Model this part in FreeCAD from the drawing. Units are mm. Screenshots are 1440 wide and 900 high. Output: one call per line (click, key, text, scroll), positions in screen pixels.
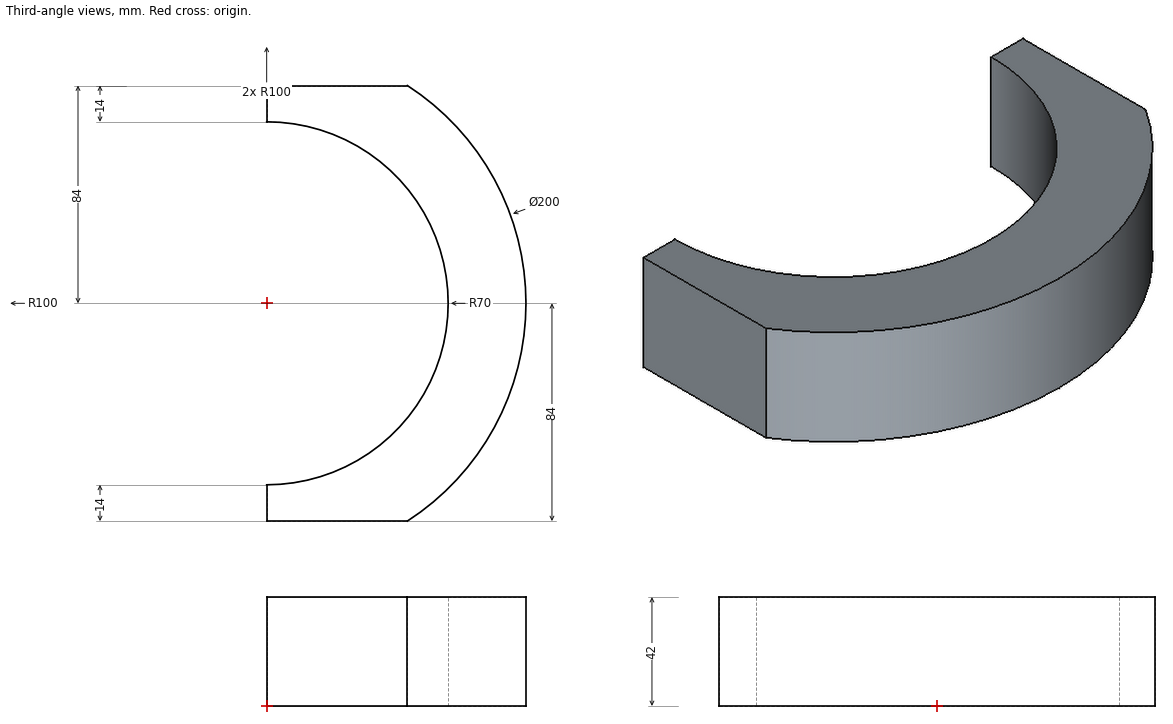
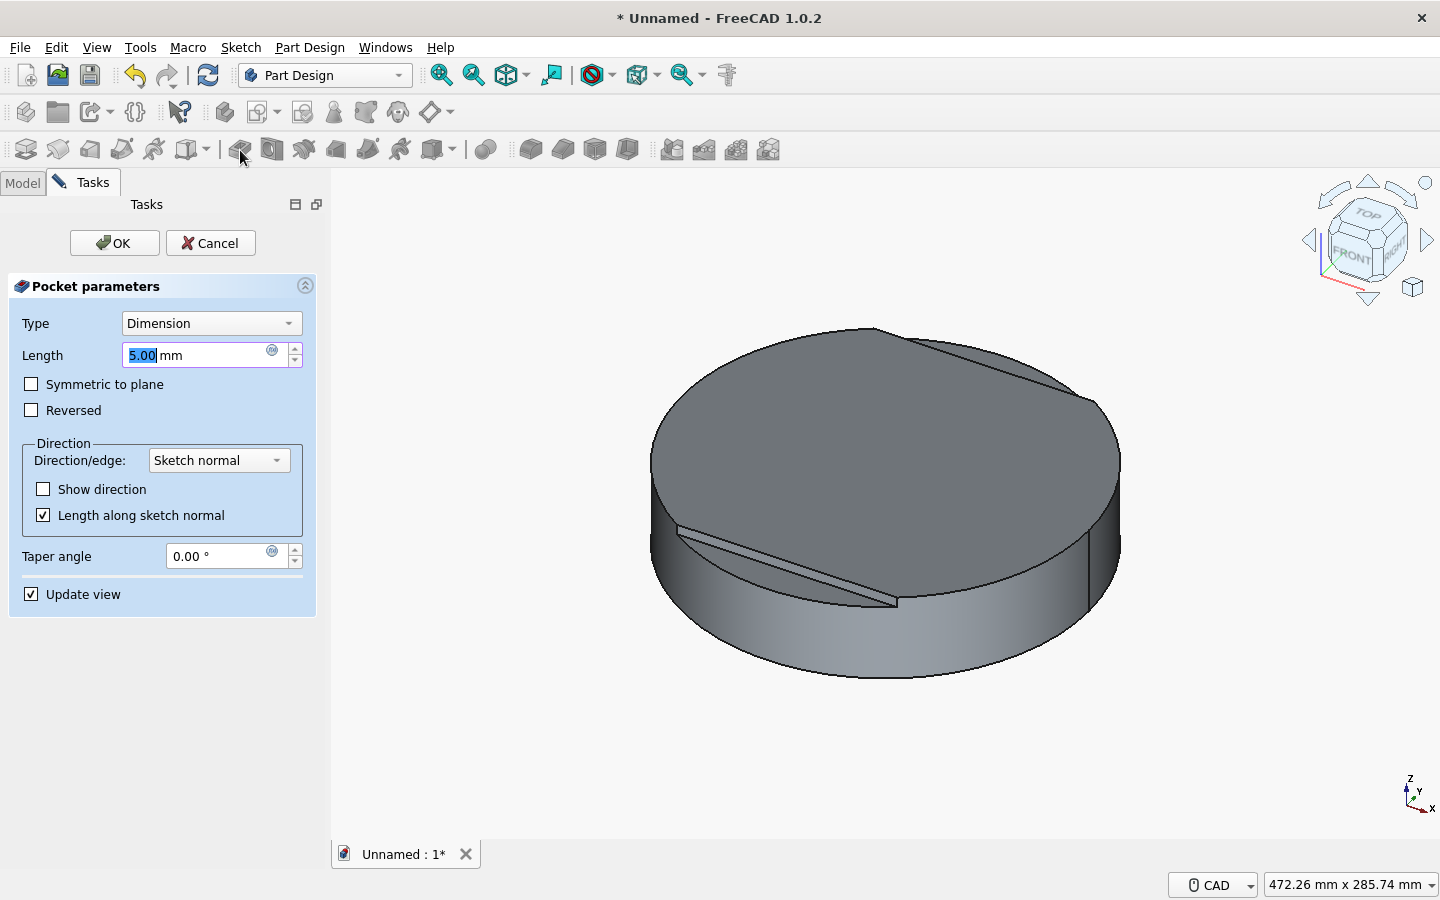
click(212, 324)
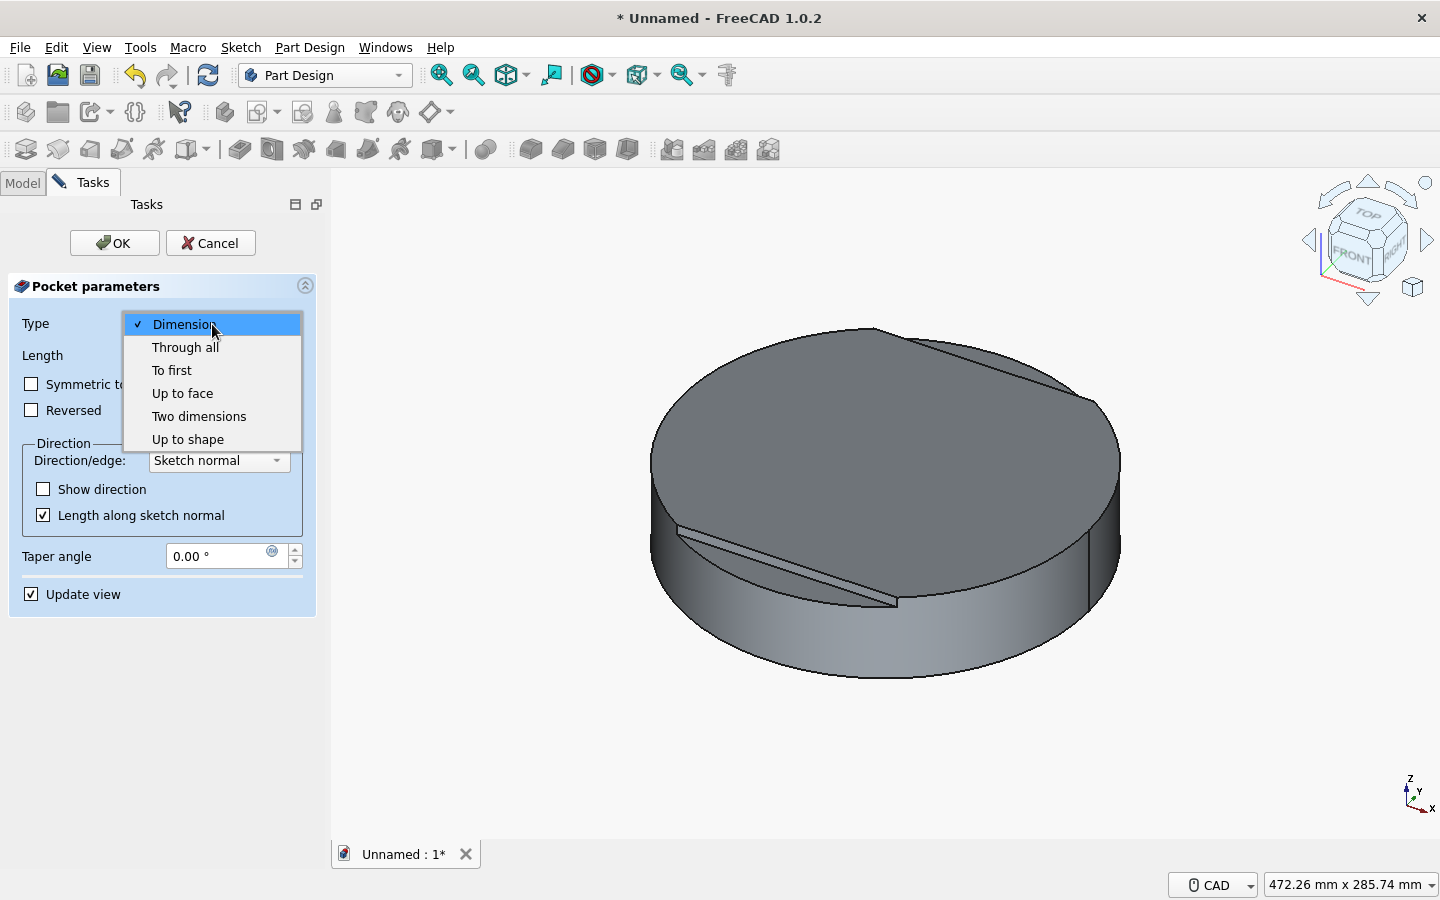
click(212, 348)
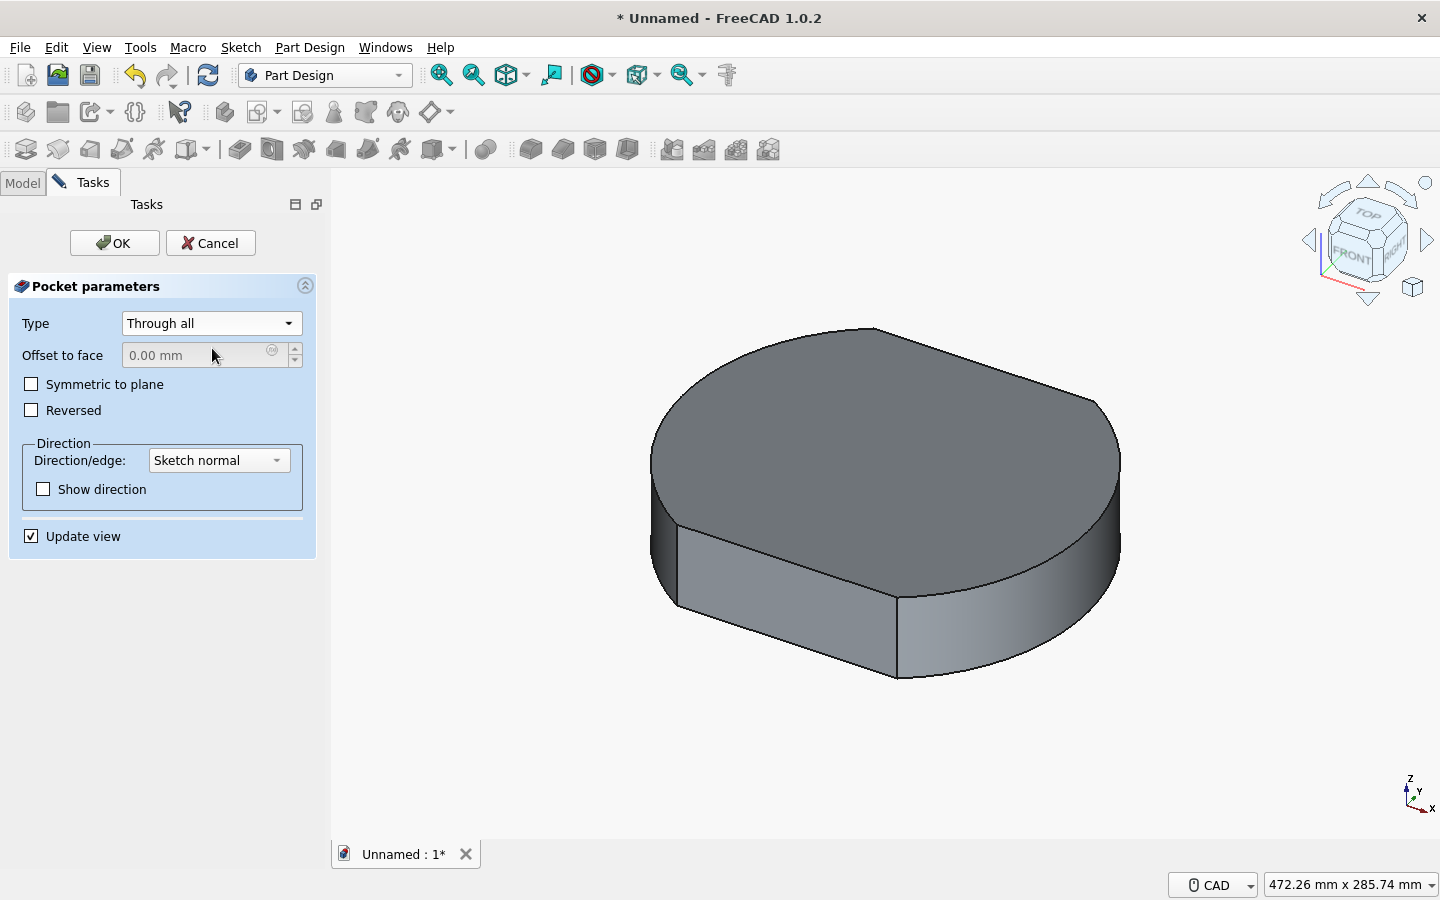
click(115, 243)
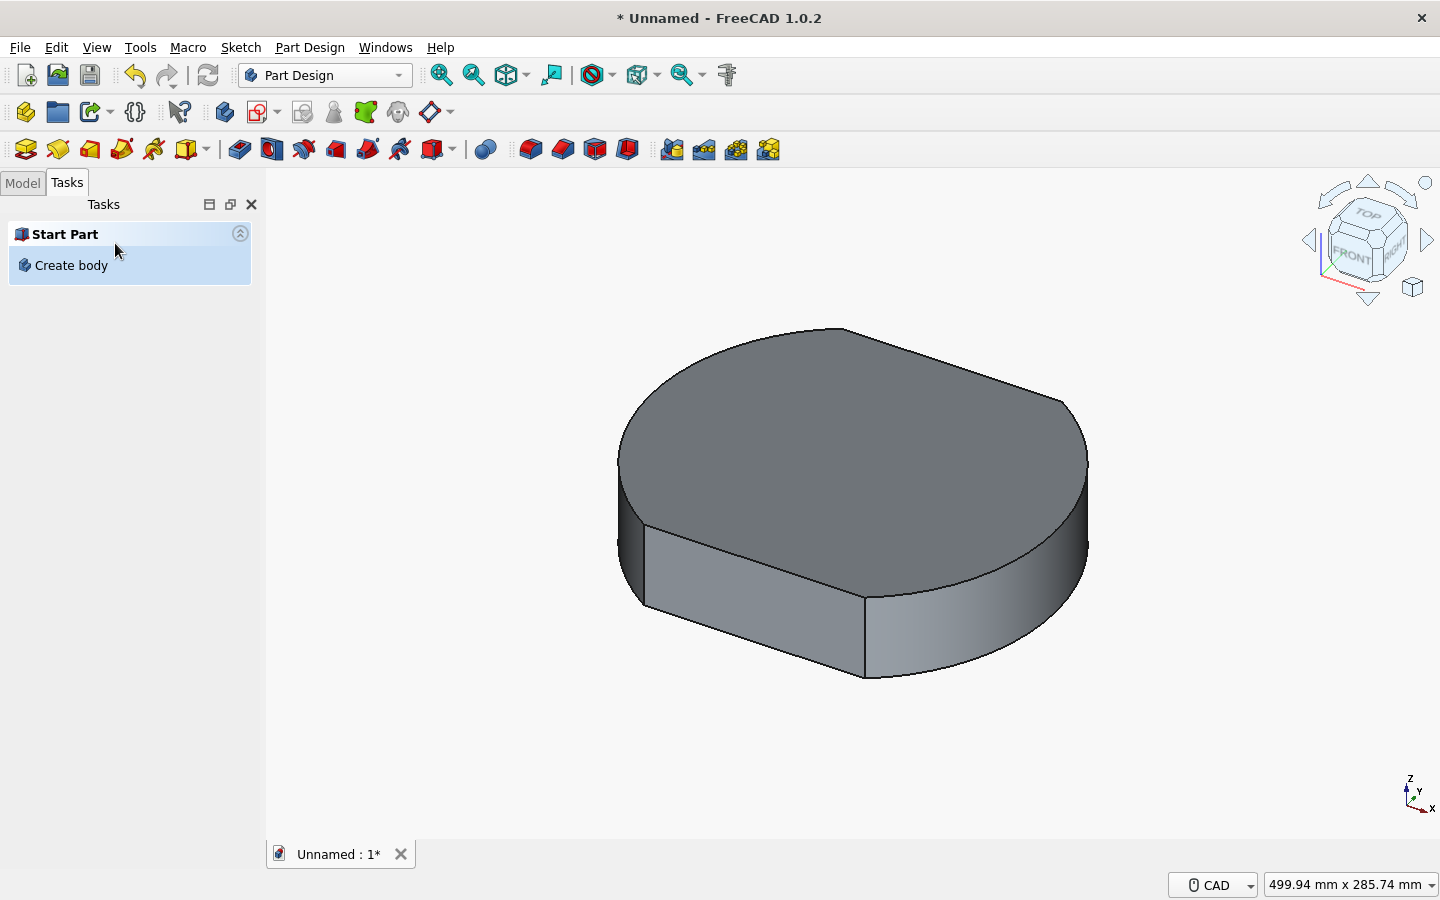
click(853, 462)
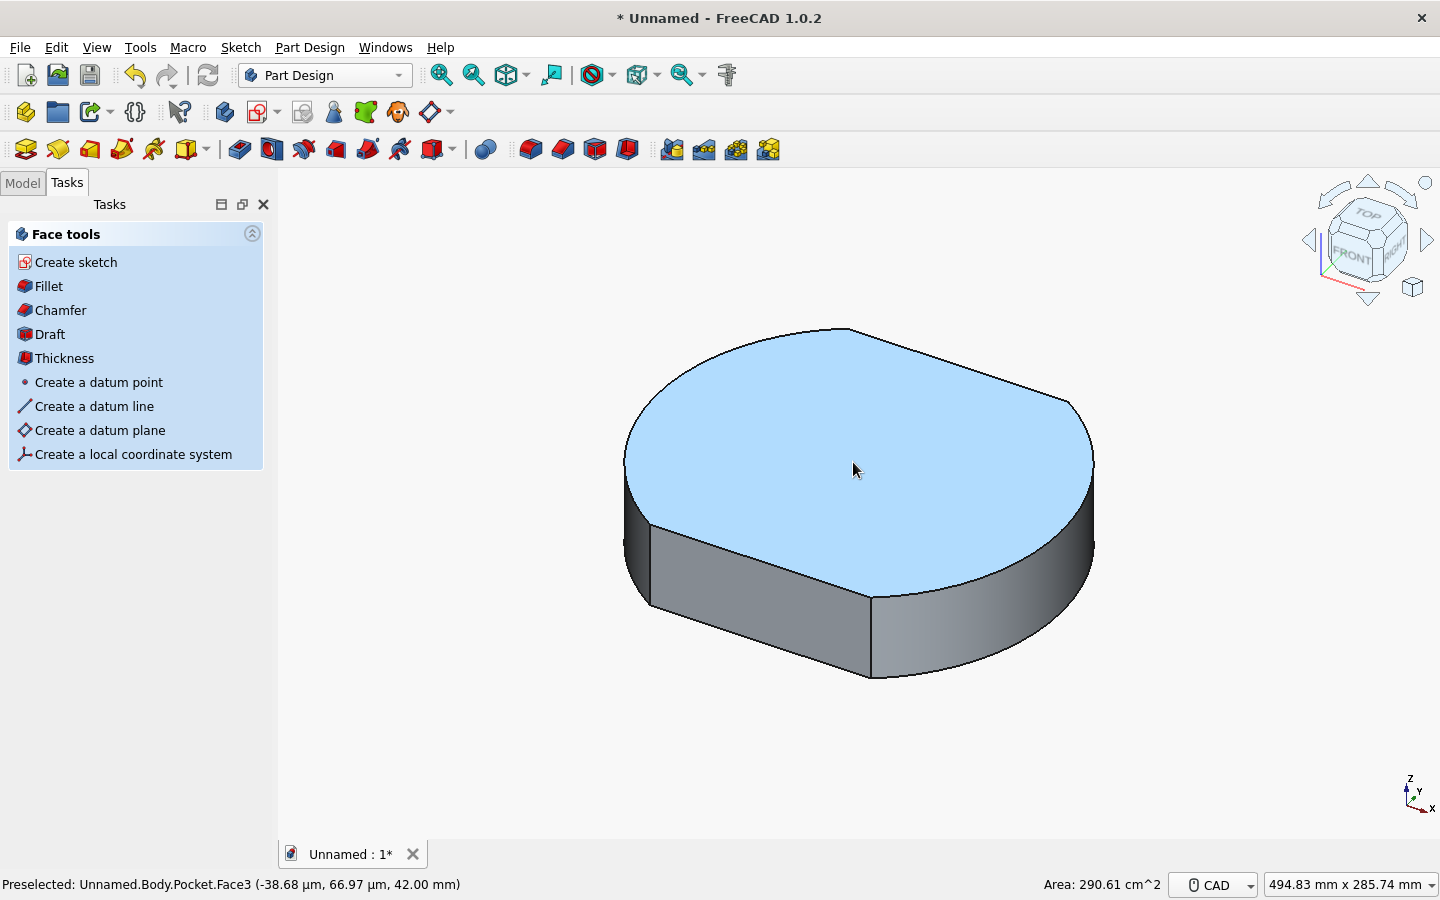
click(258, 112)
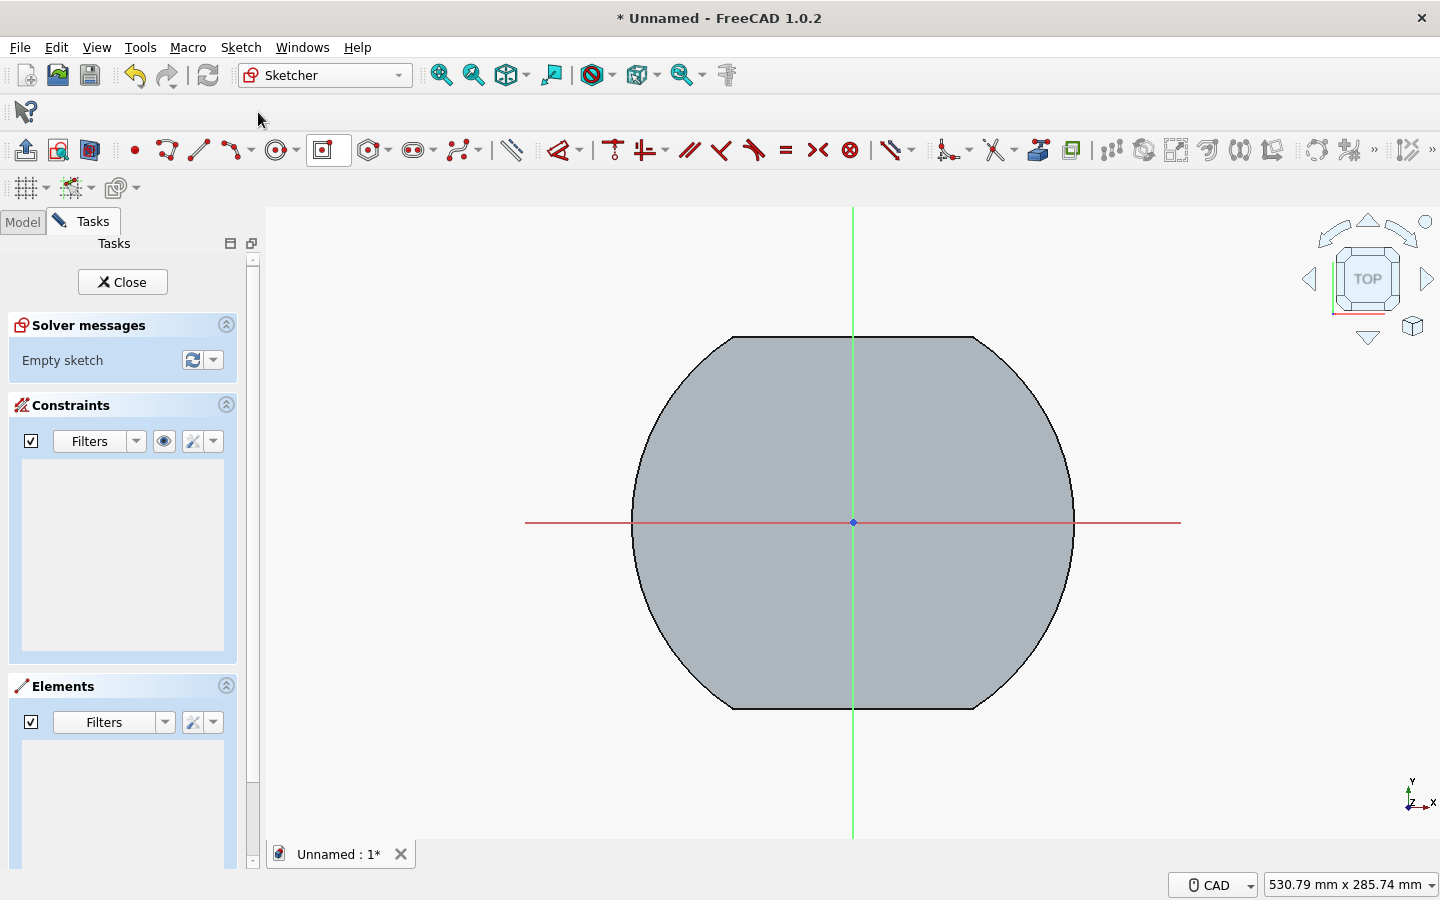
click(168, 150)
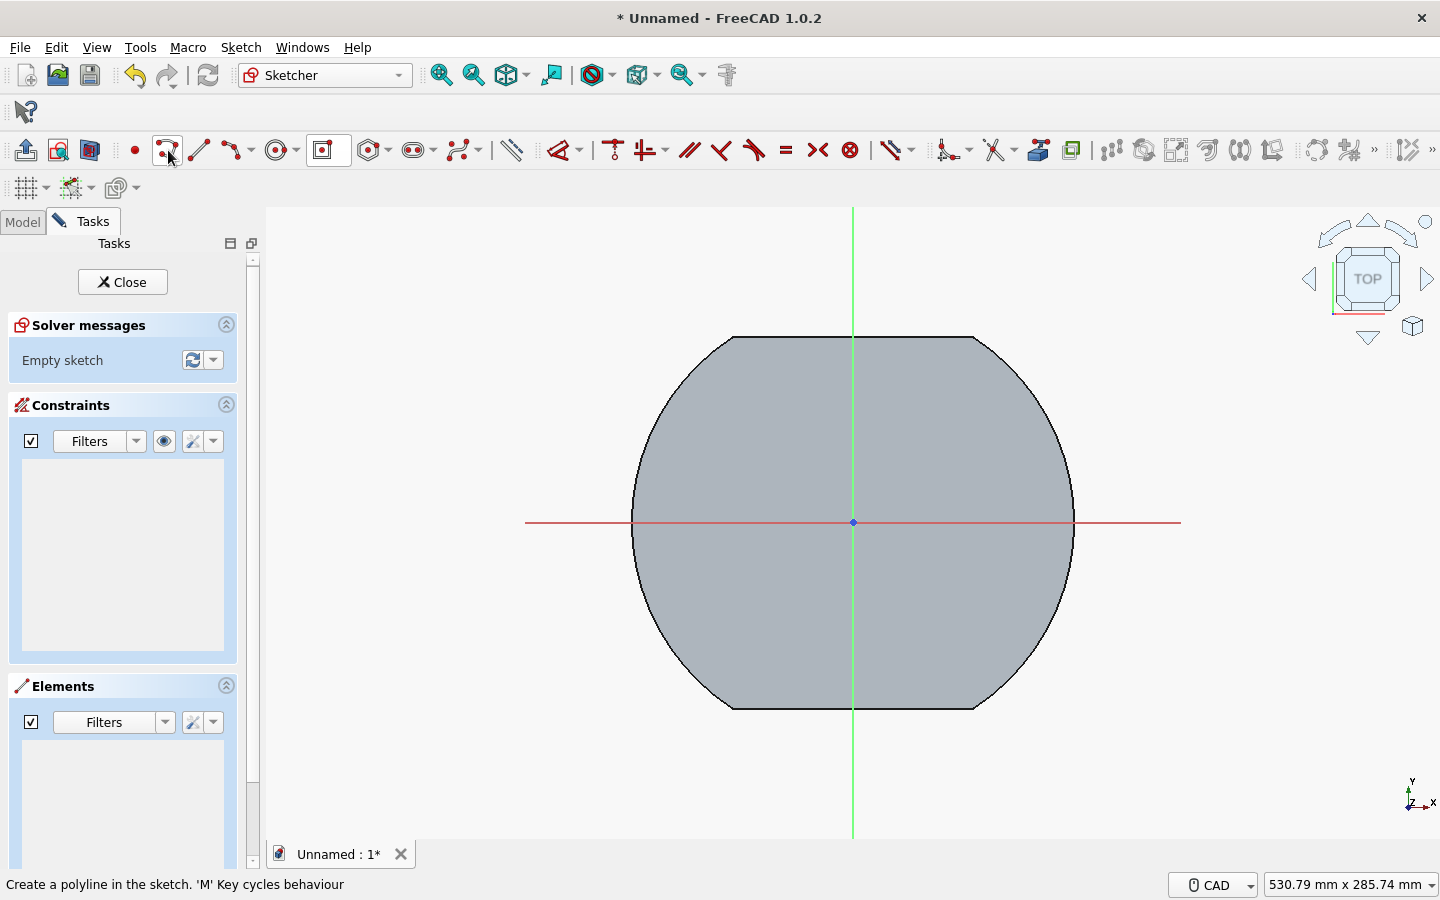
click(853, 368)
click(844, 337)
click(733, 337)
right_click(733, 337)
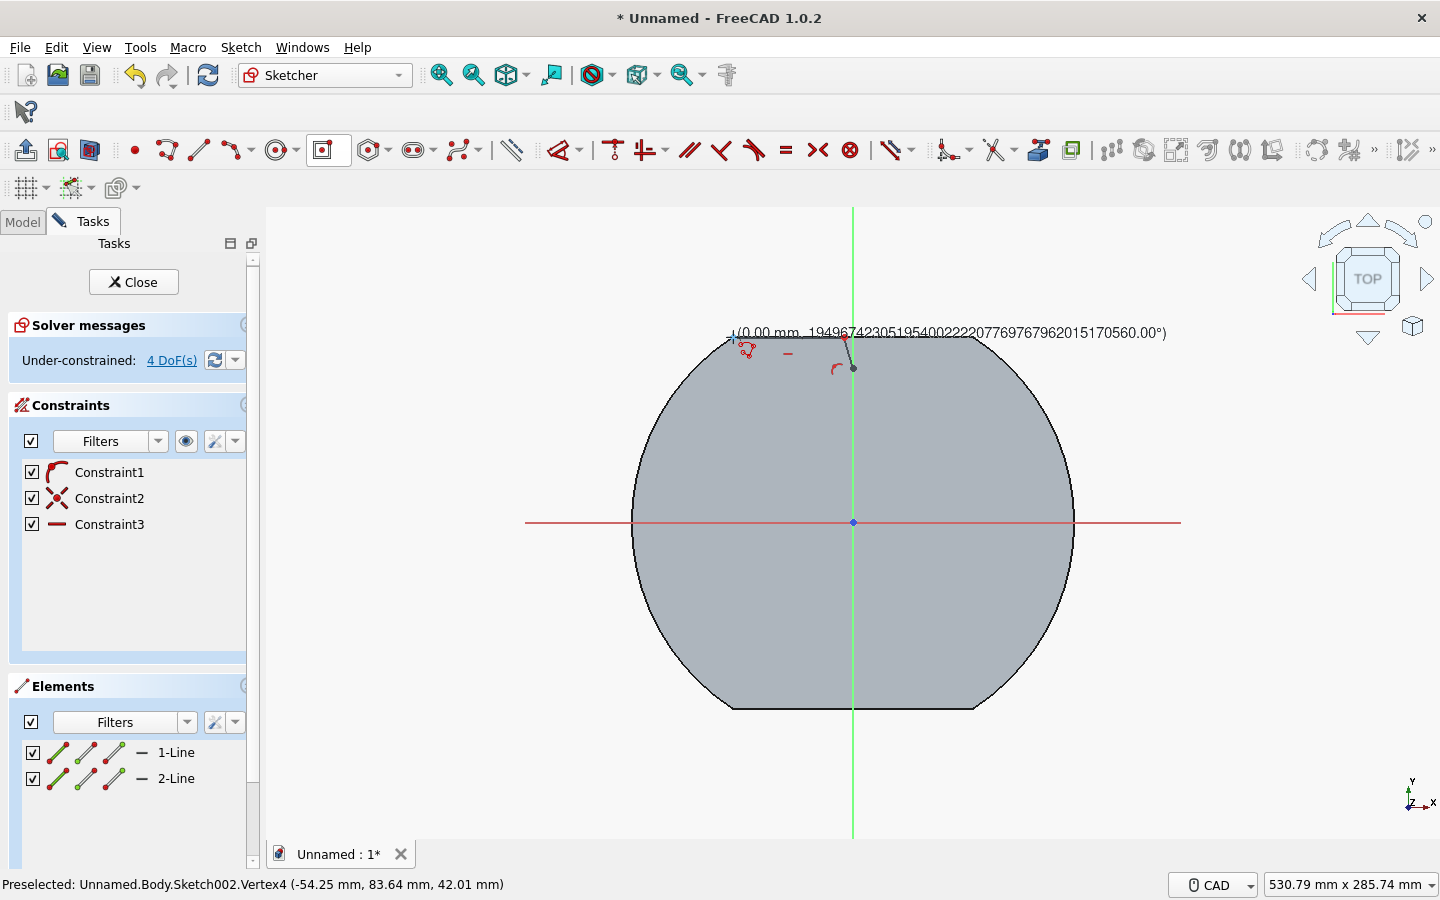
click(733, 709)
click(853, 709)
click(844, 678)
right_click(844, 678)